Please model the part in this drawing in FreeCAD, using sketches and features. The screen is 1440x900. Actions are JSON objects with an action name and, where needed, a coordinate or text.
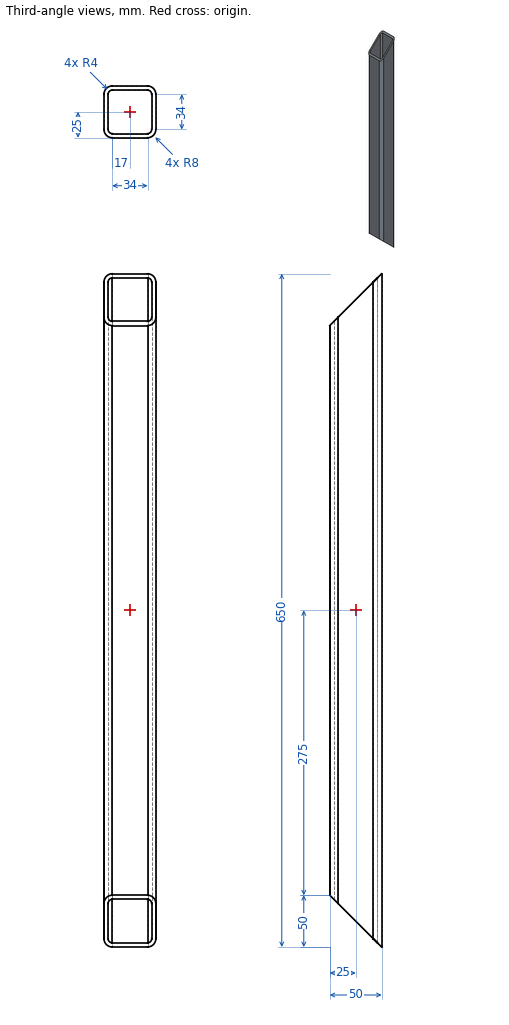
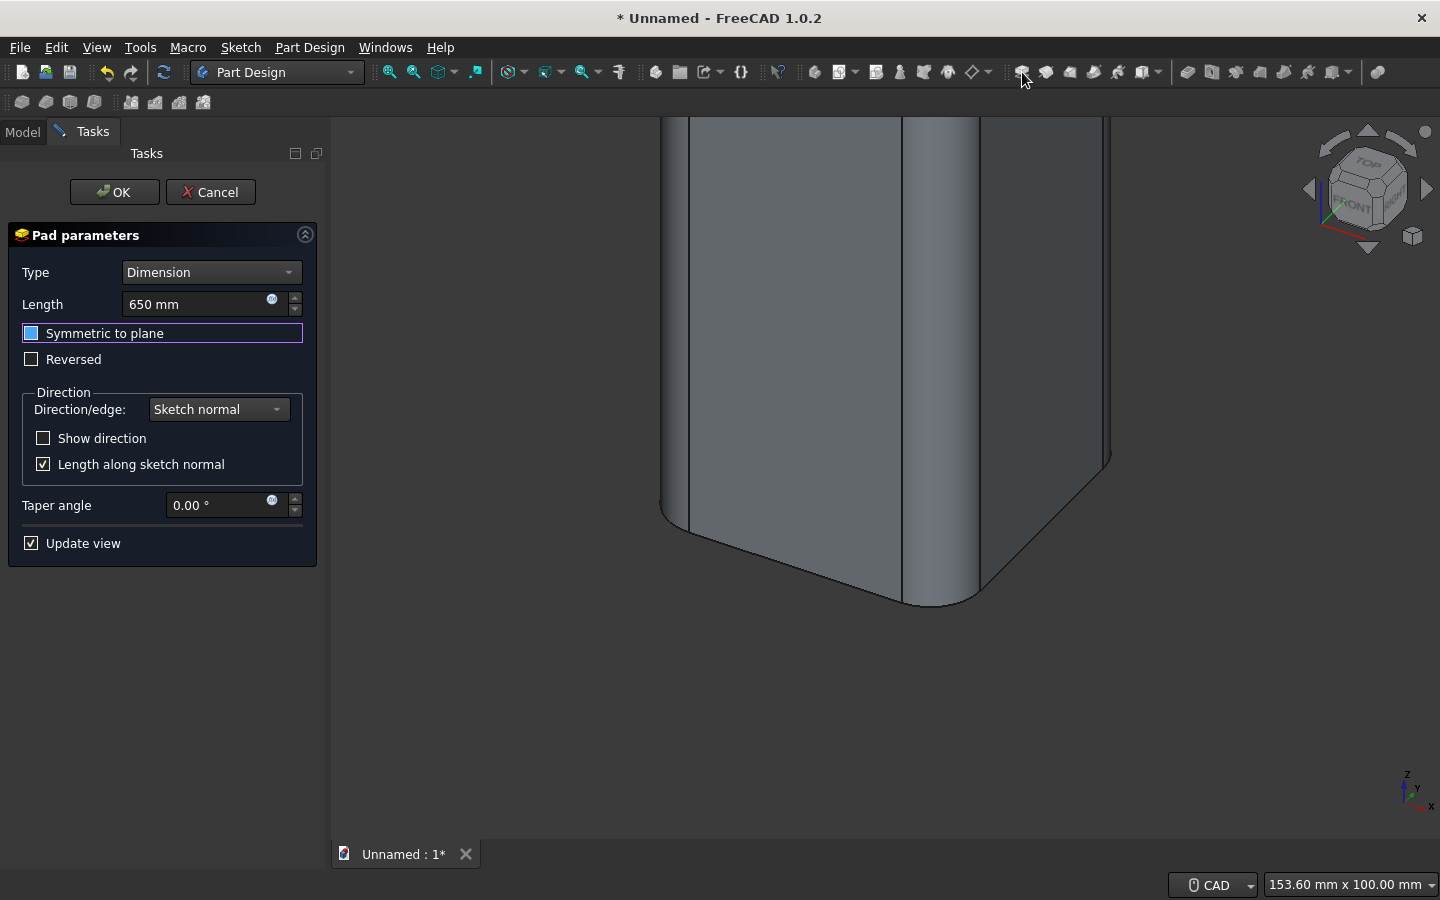
{"action": "left_click", "coordinate": [30, 333]}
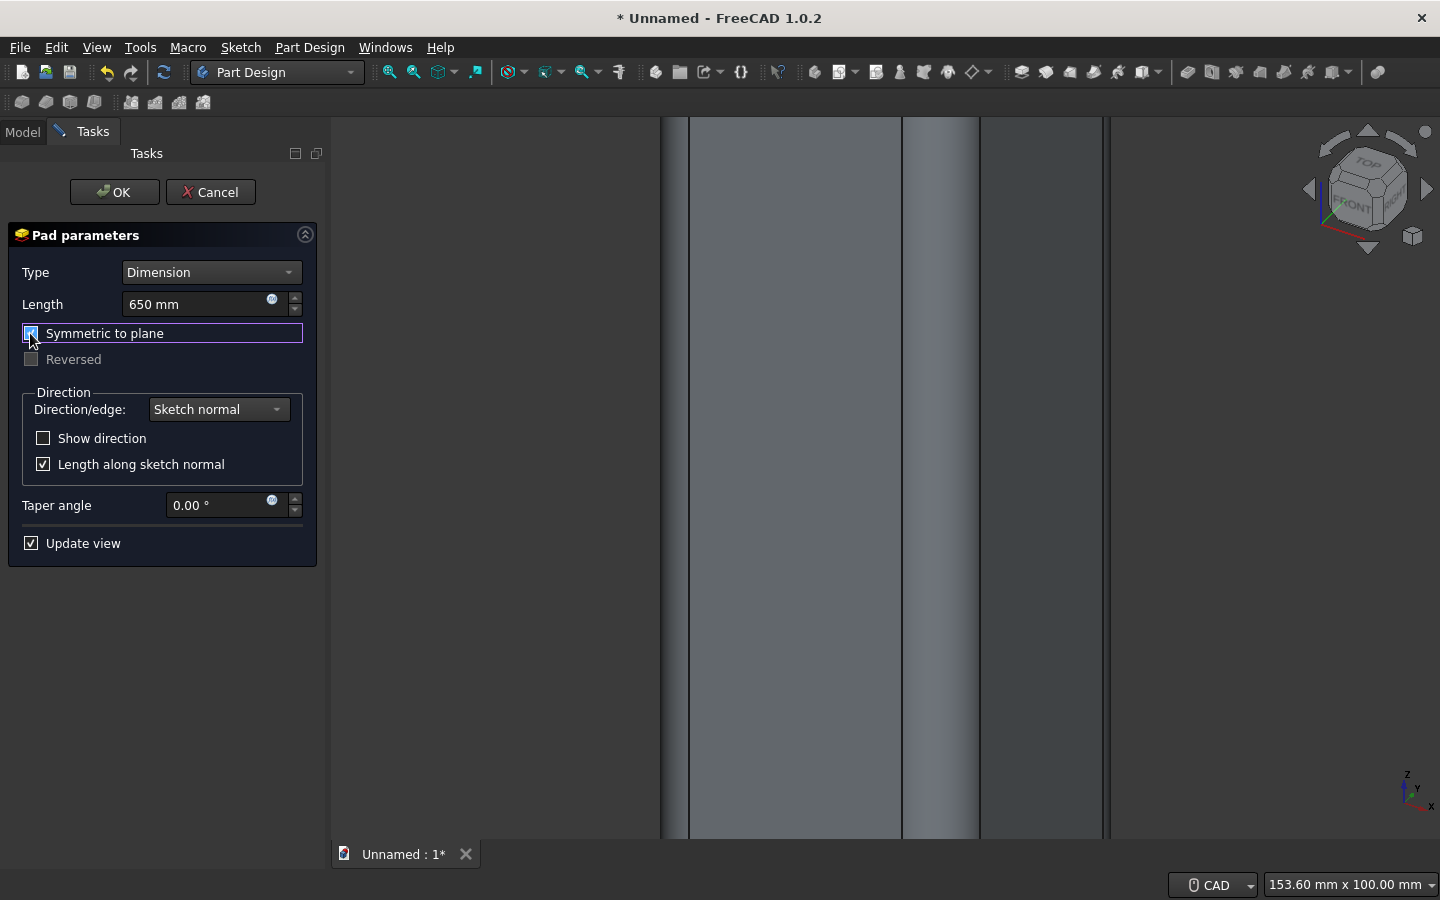
{"action": "left_click", "coordinate": [115, 192]}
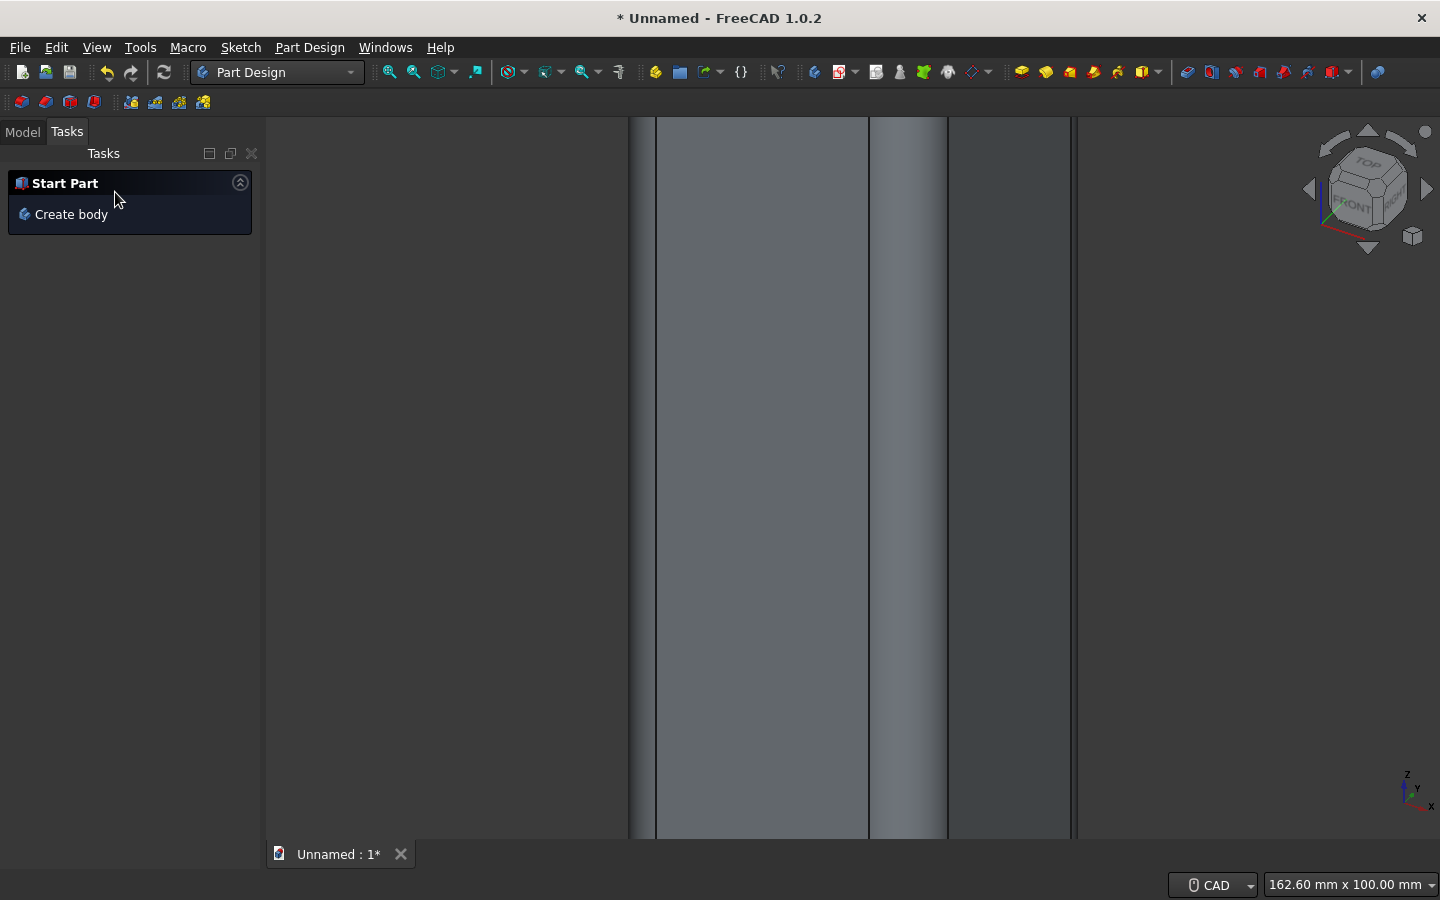
{"action": "left_click", "coordinate": [390, 72]}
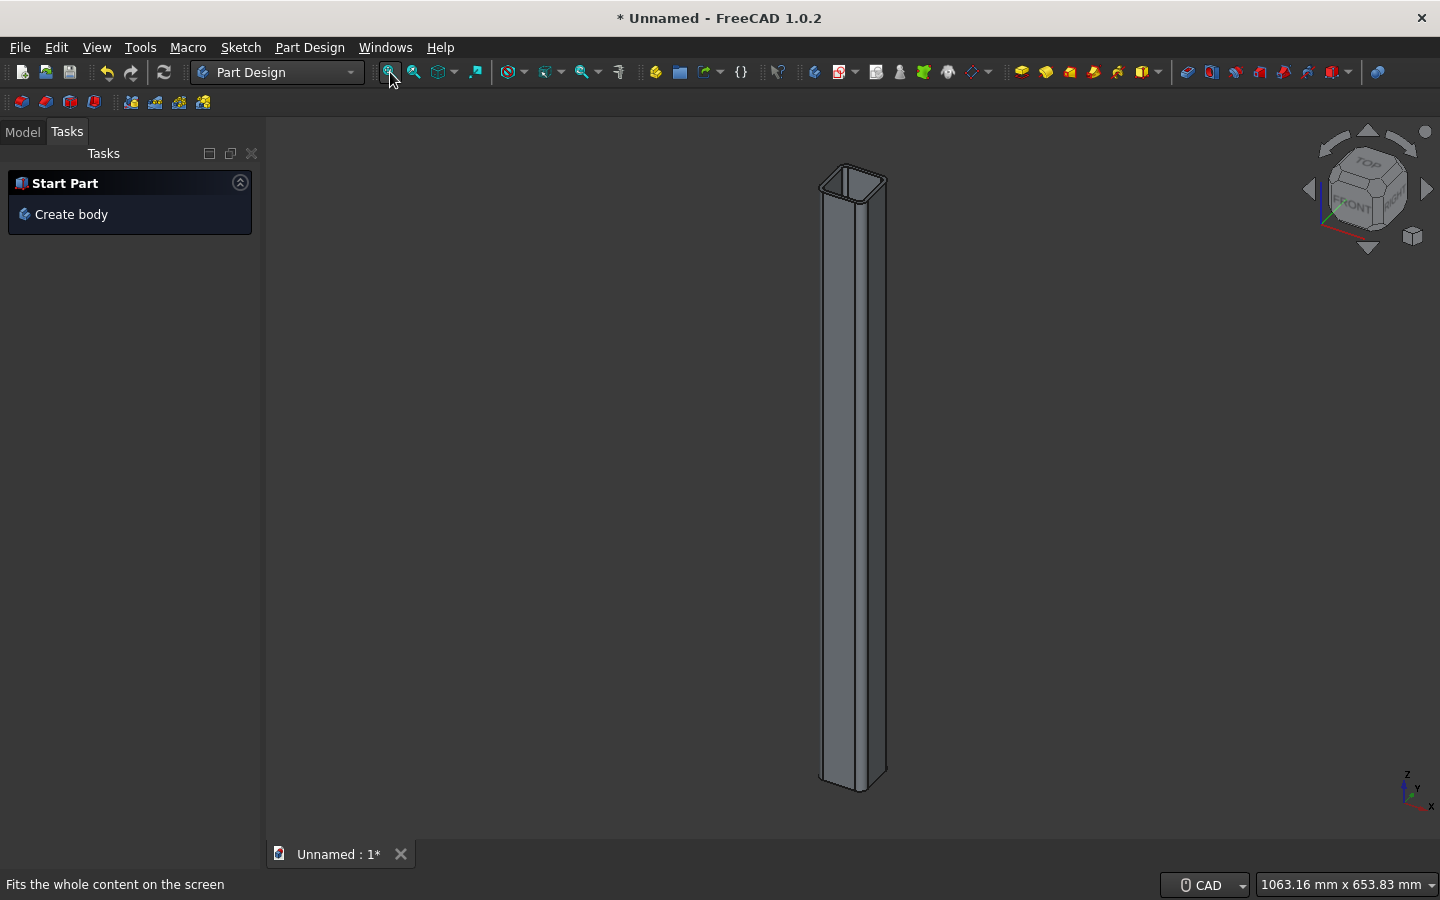
{"action": "key", "text": "6"}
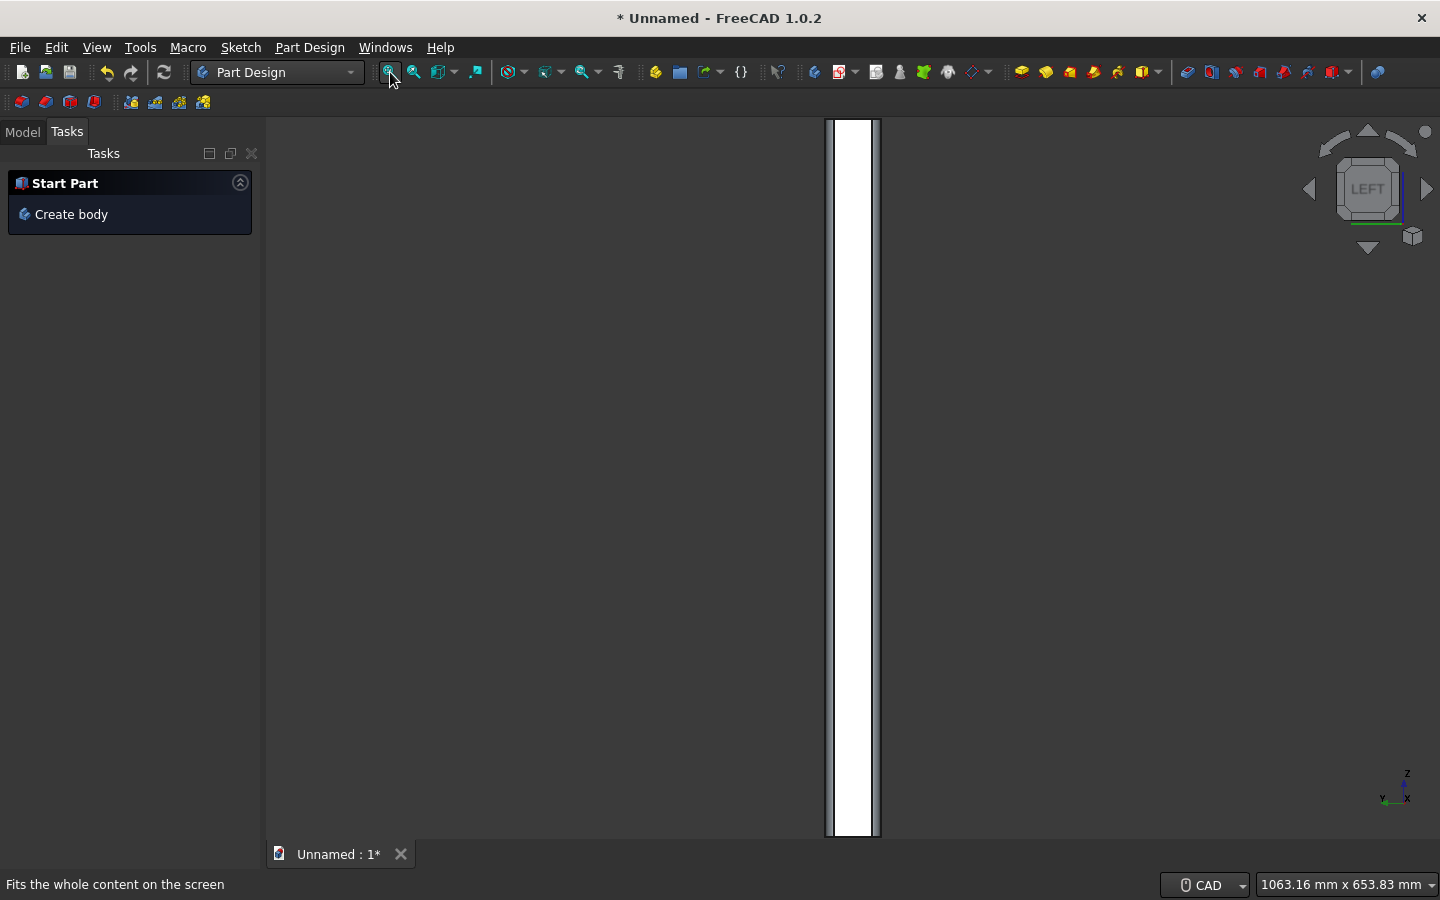
{"action": "left_click", "coordinate": [853, 169]}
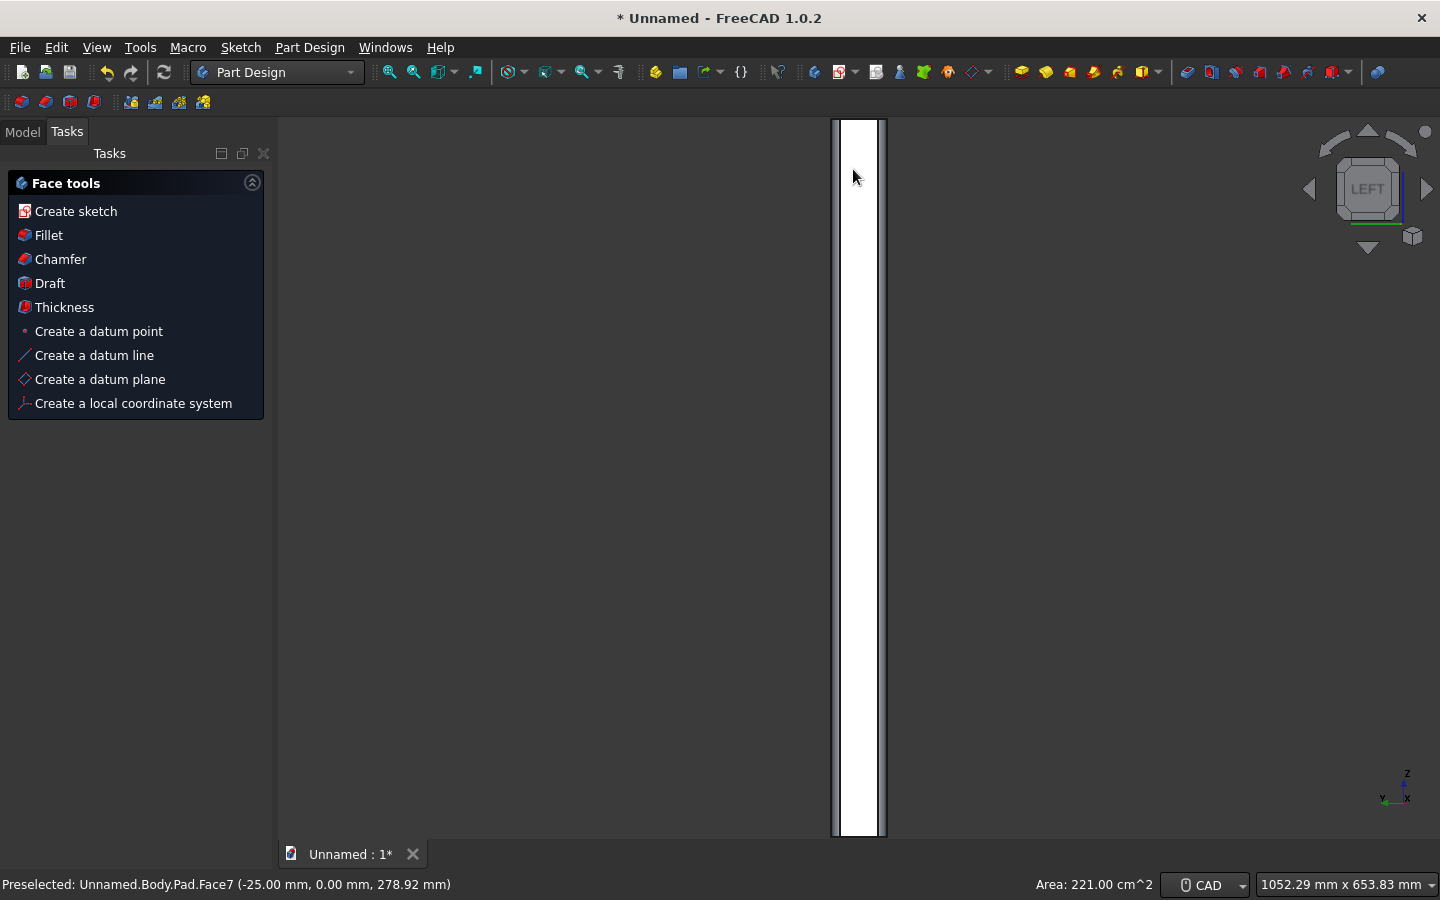
{"action": "left_click", "coordinate": [840, 72]}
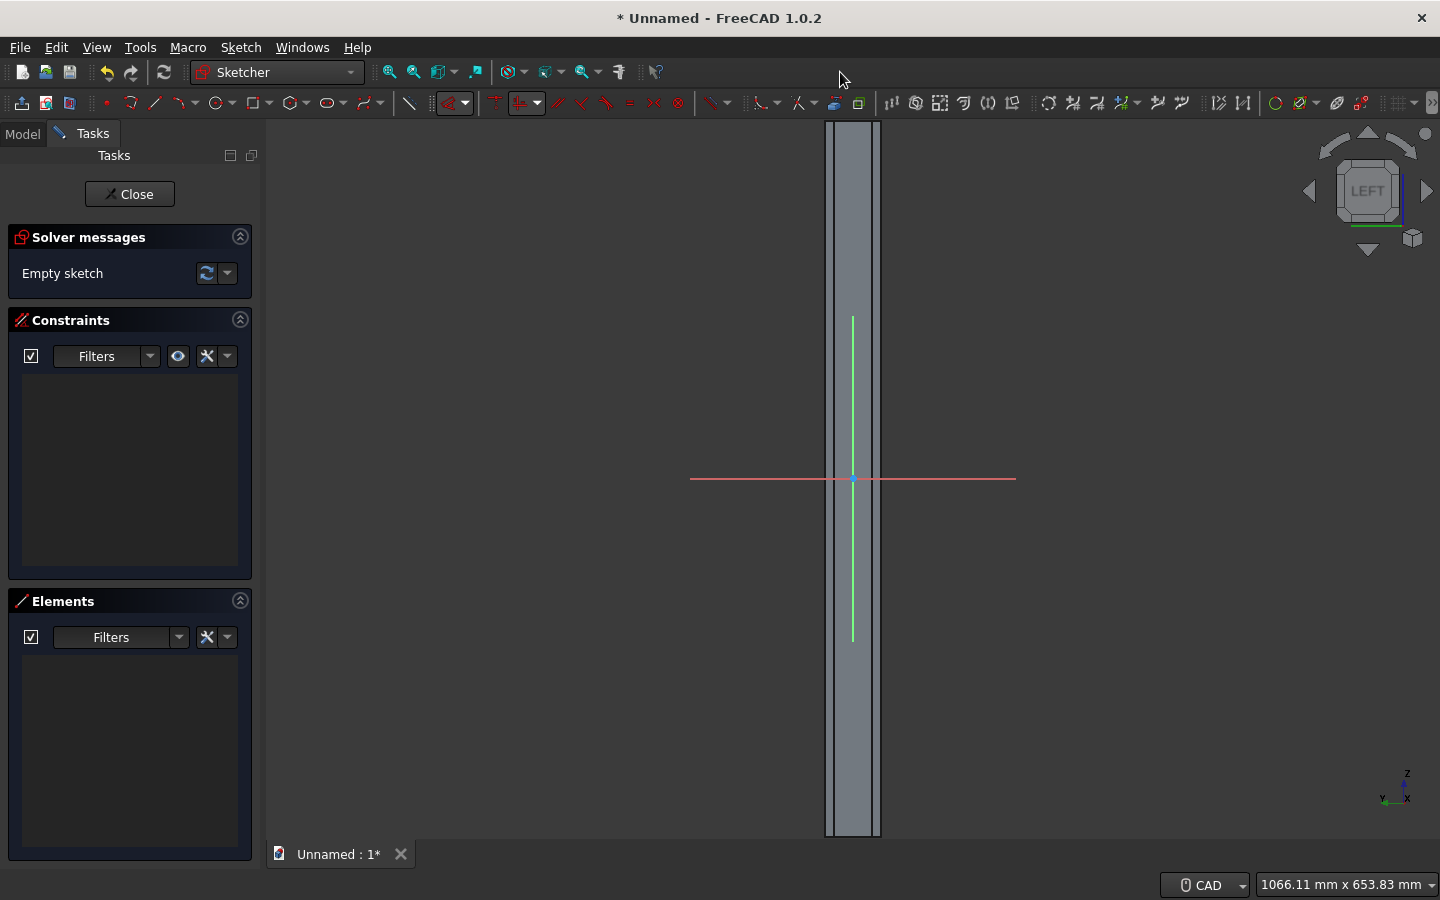
{"action": "scroll", "coordinate": [784, 479], "scroll_direction": "down", "scroll_amount": 5}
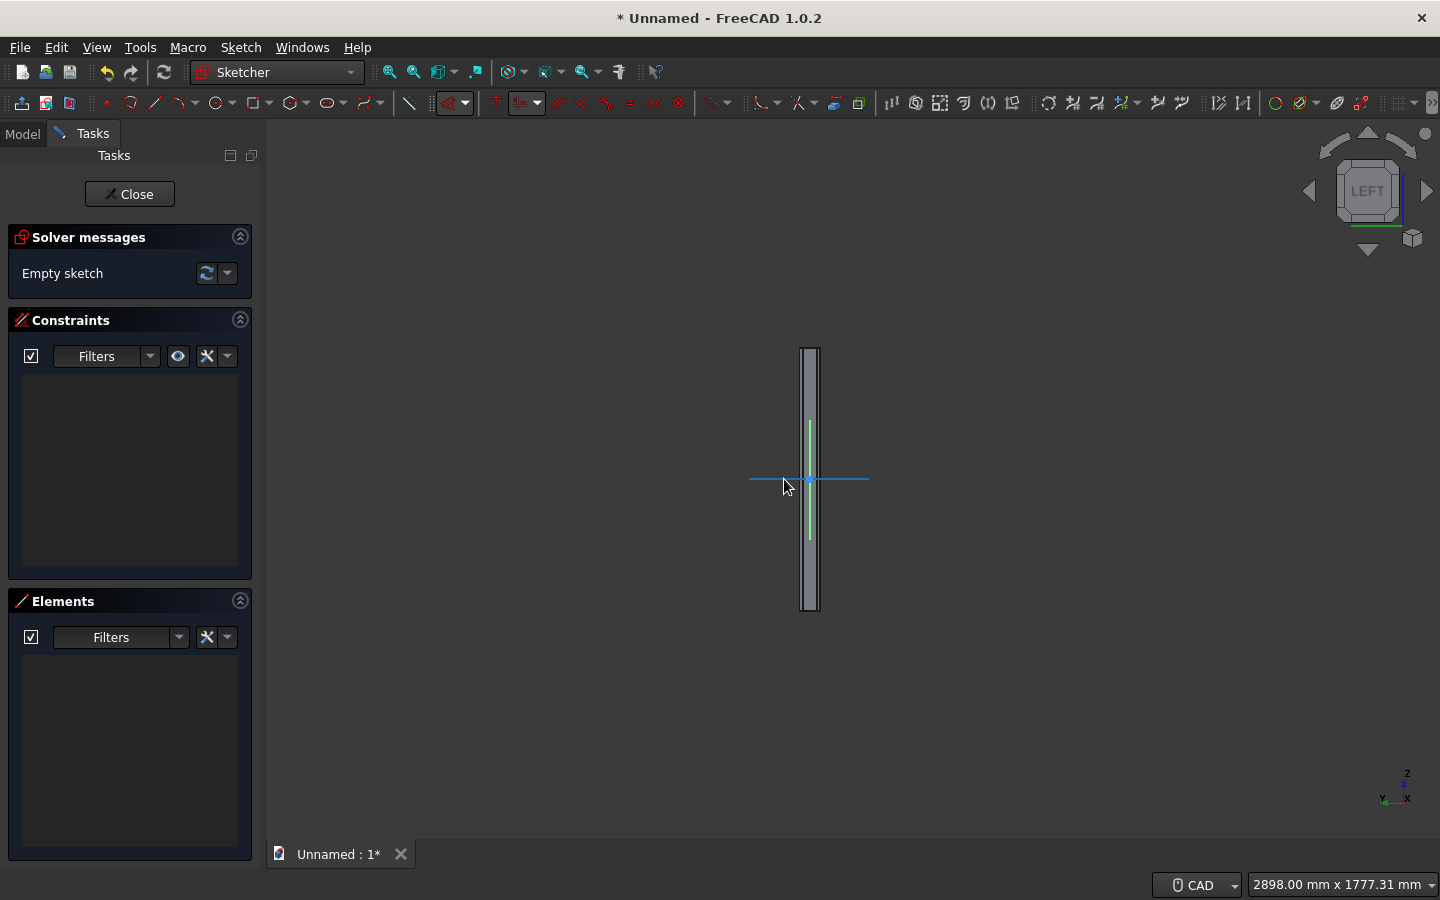
{"action": "scroll", "coordinate": [811, 607], "scroll_direction": "up", "scroll_amount": 15}